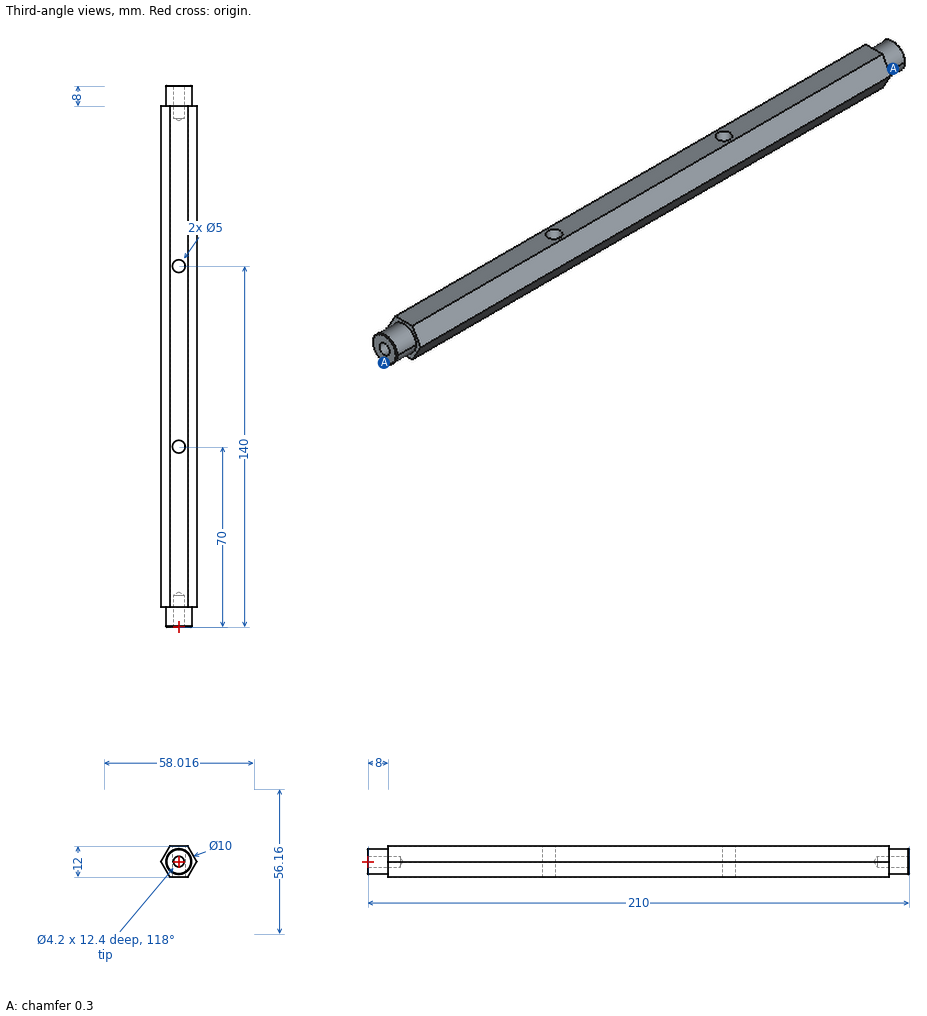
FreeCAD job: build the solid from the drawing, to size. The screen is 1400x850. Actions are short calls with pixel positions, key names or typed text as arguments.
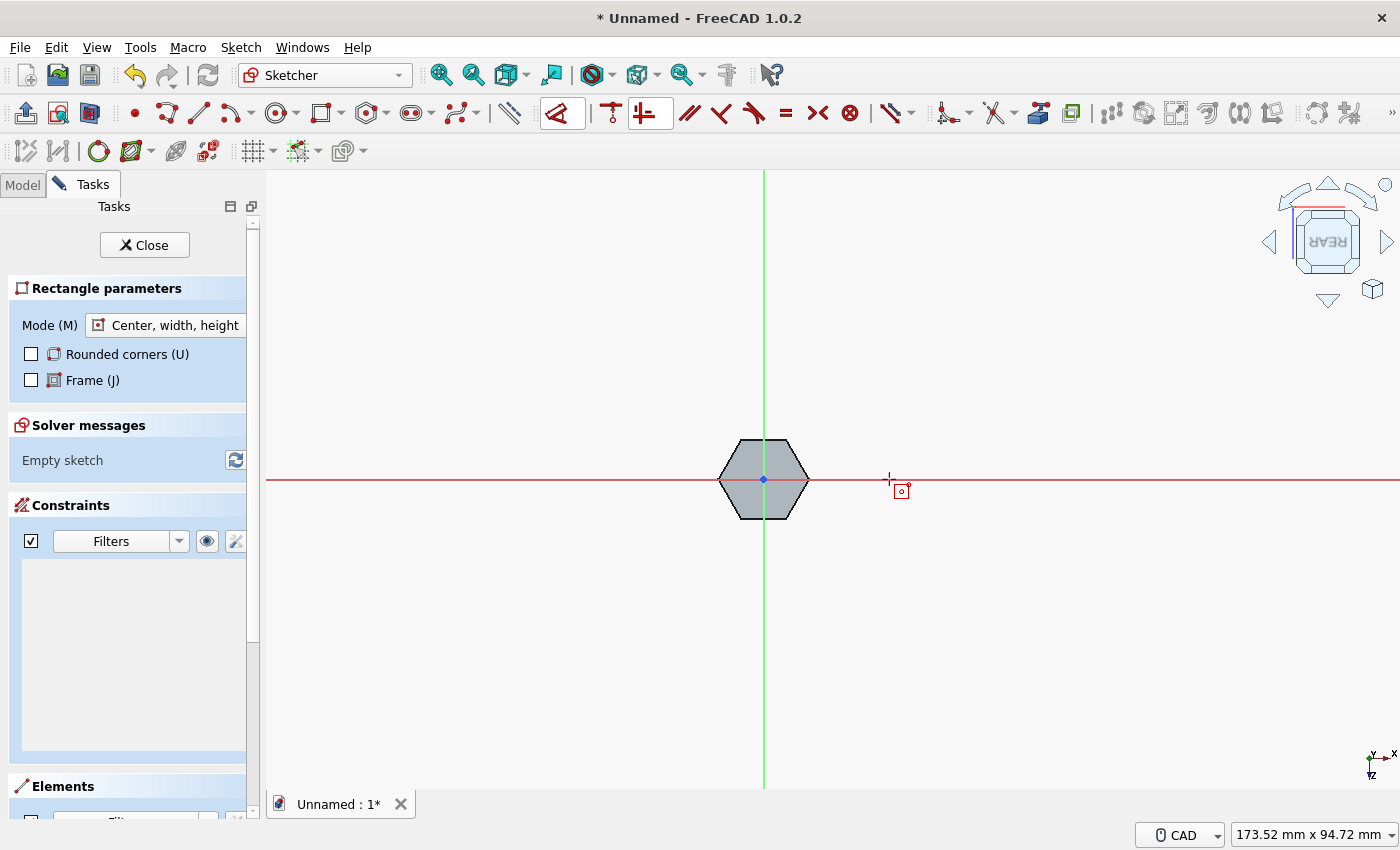
click(764, 479)
click(953, 296)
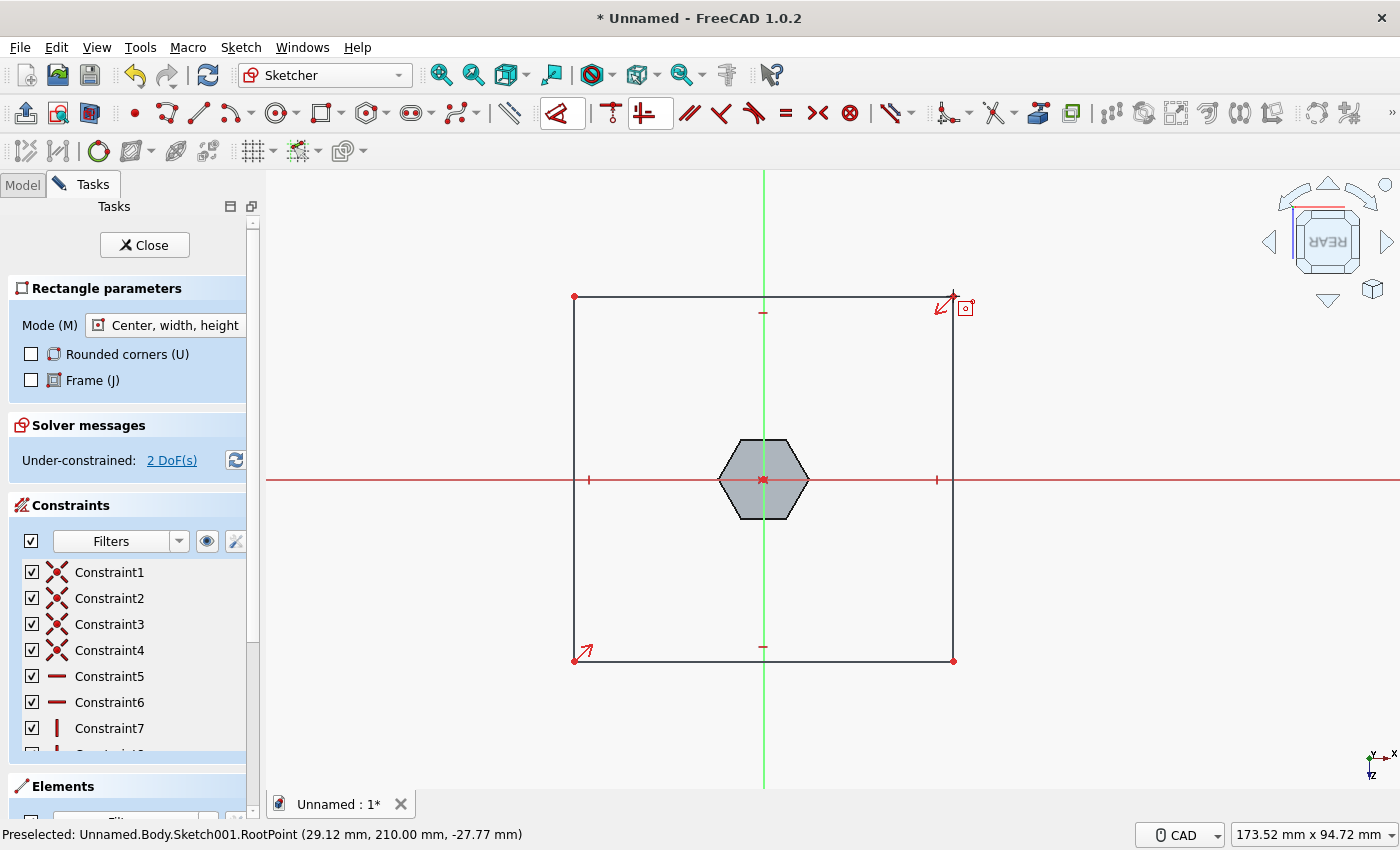
key(g)
key(c)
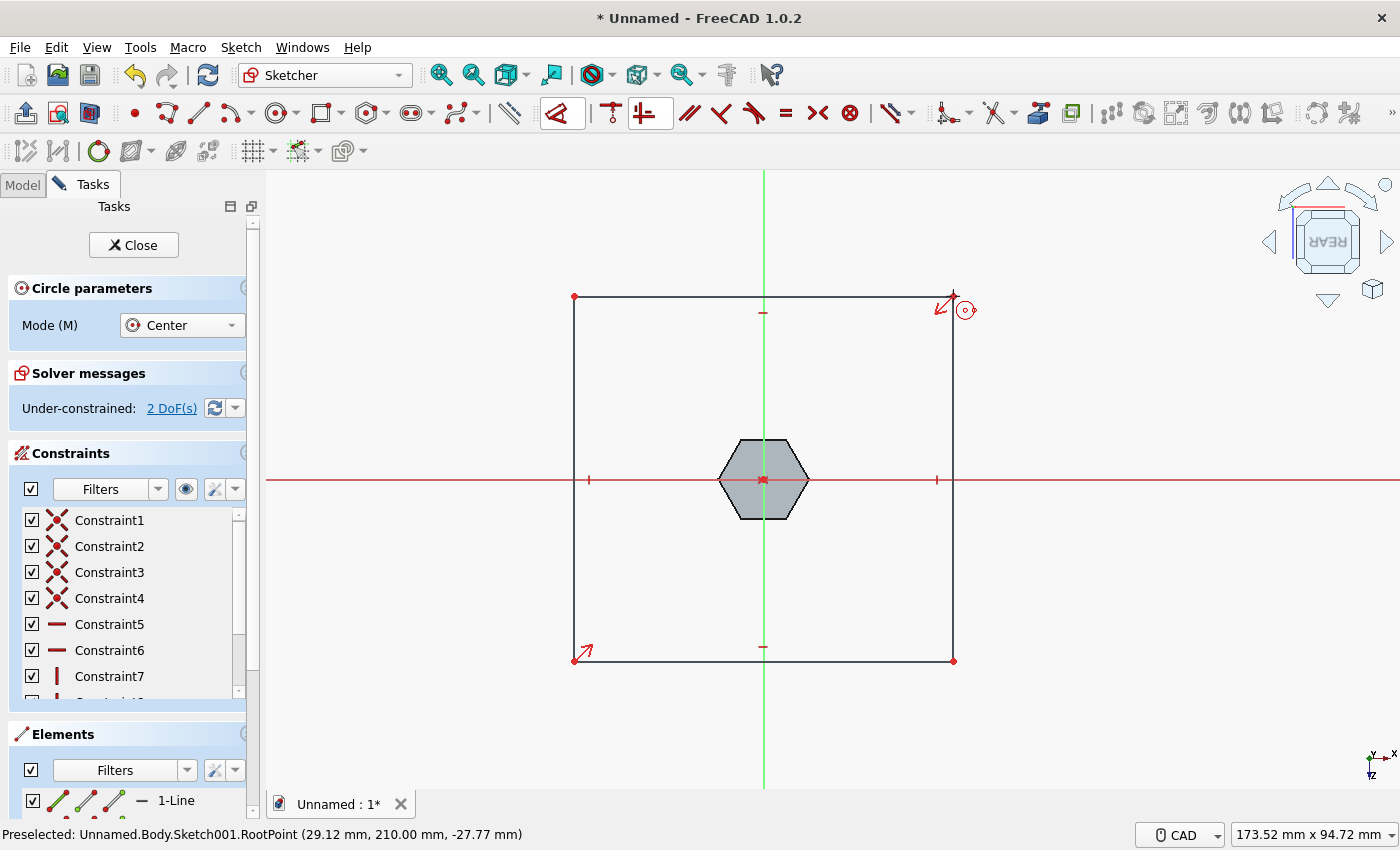
click(764, 479)
click(787, 456)
key(Escape)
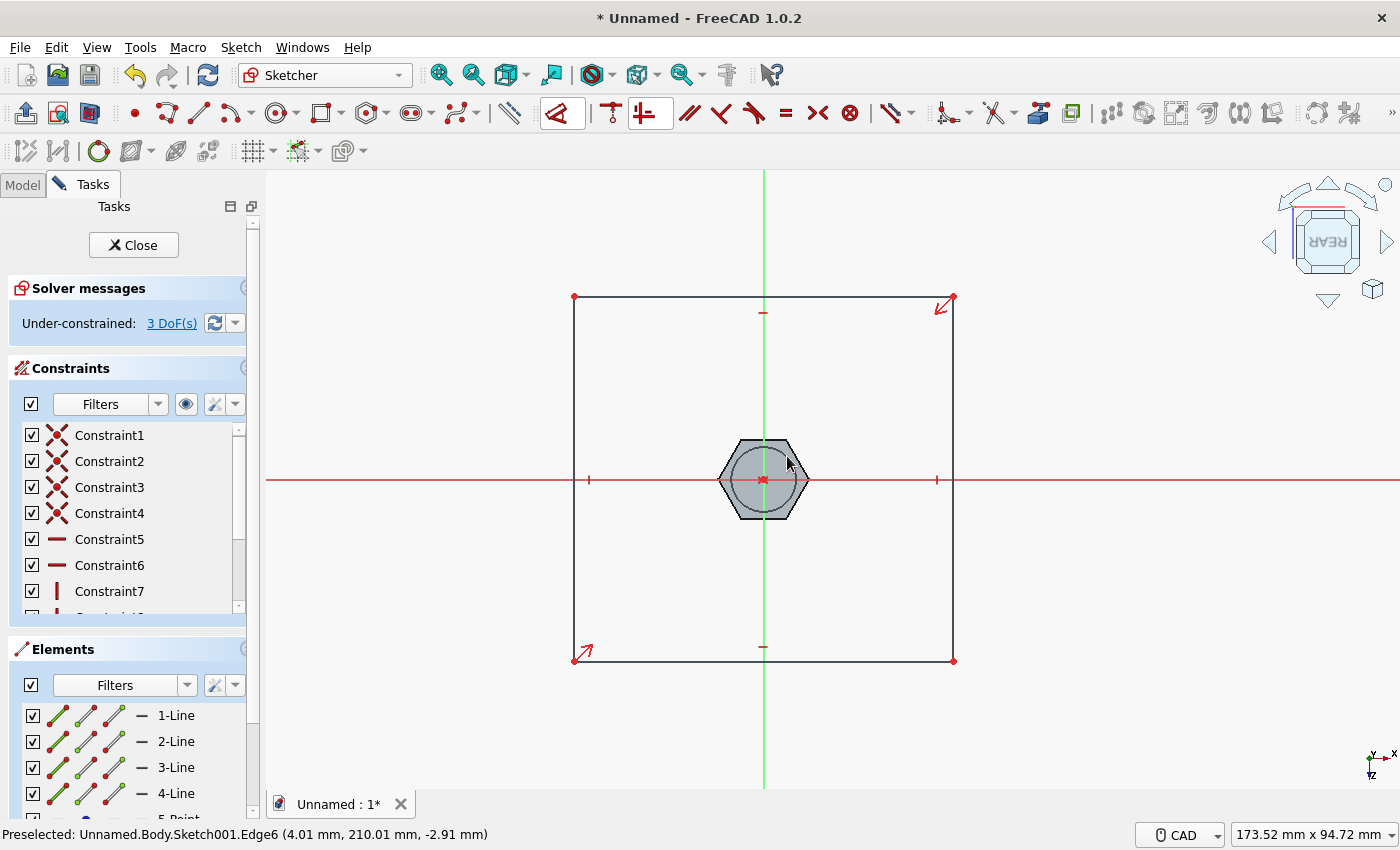
click(787, 457)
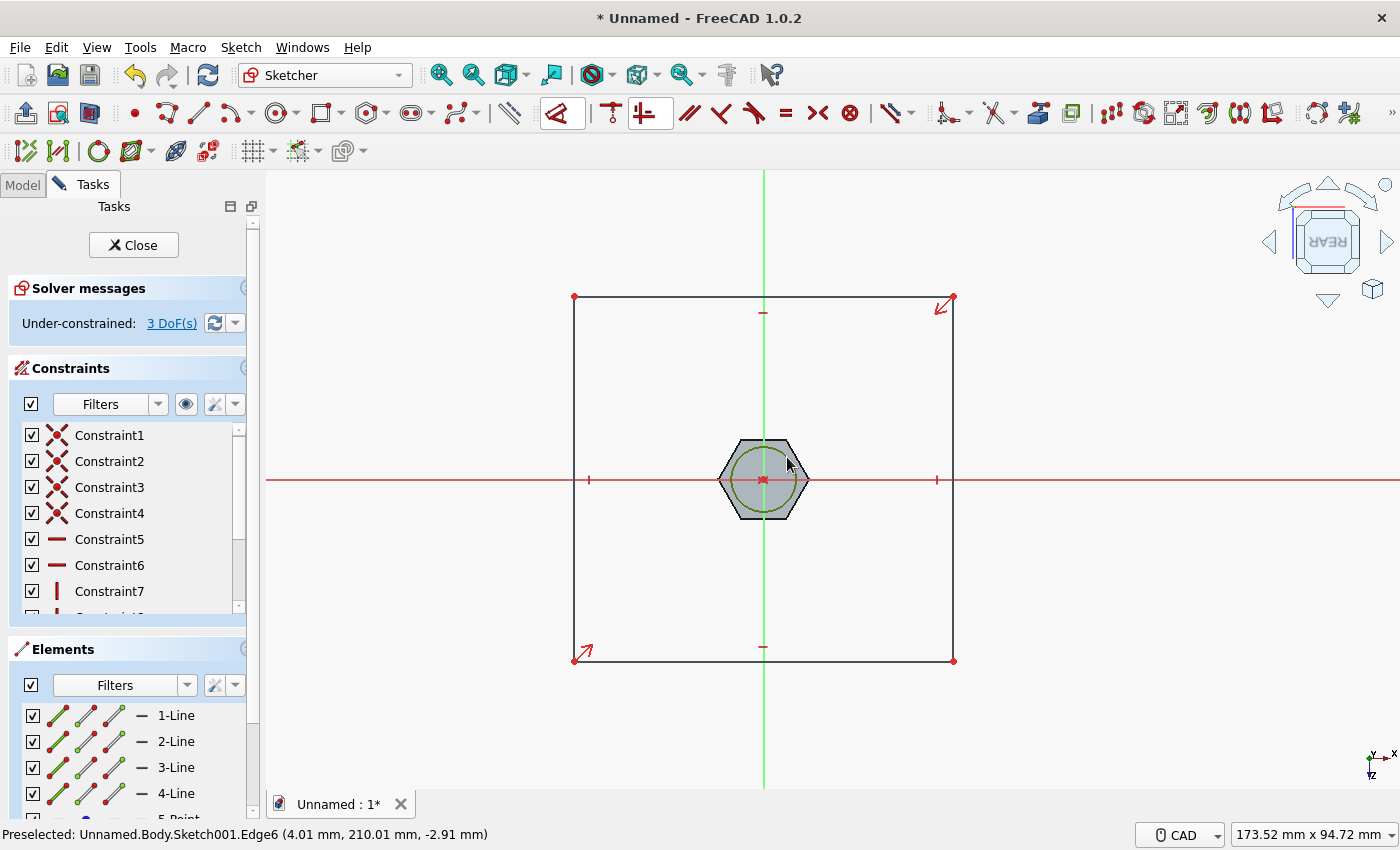
click(580, 114)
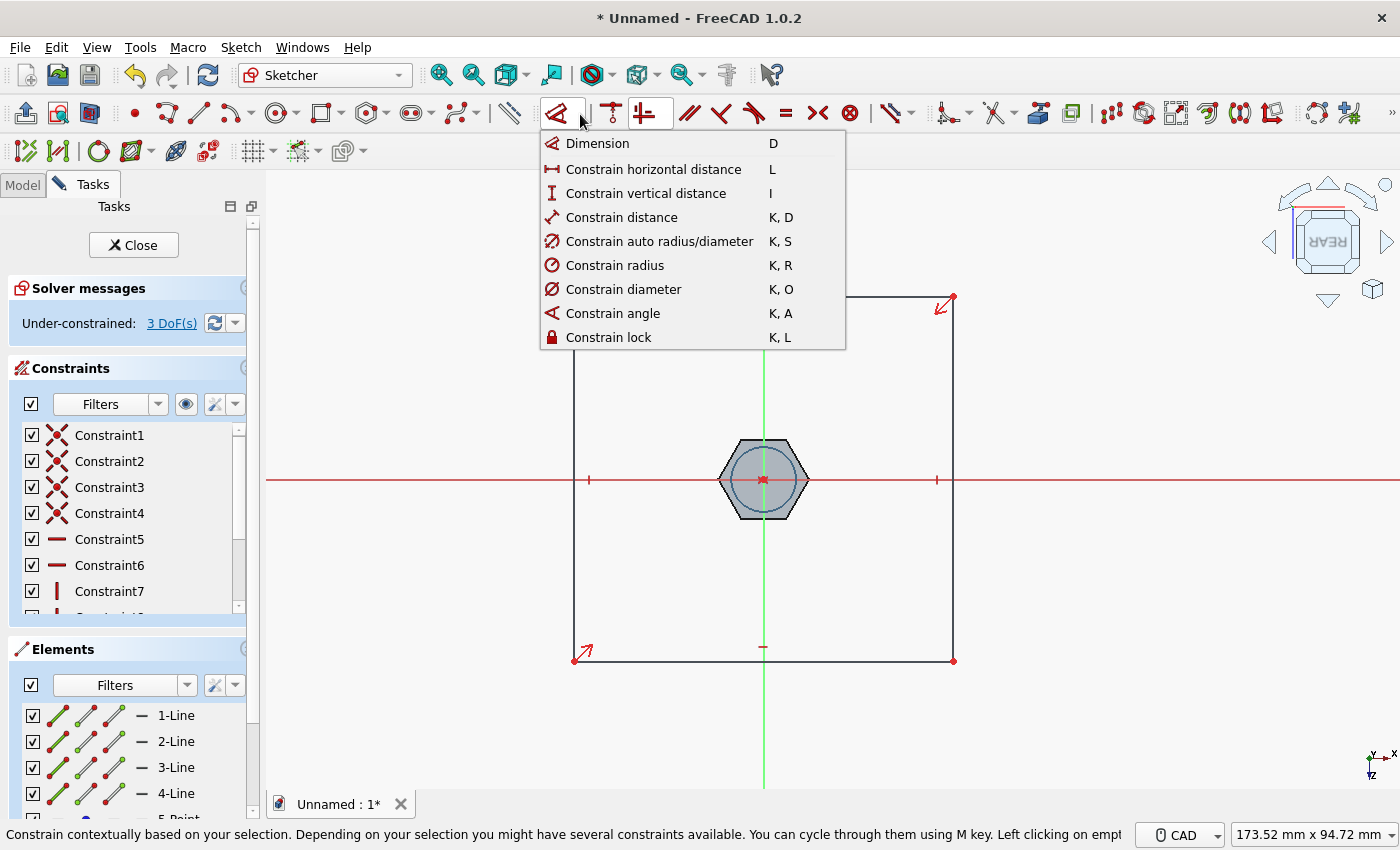
click(693, 289)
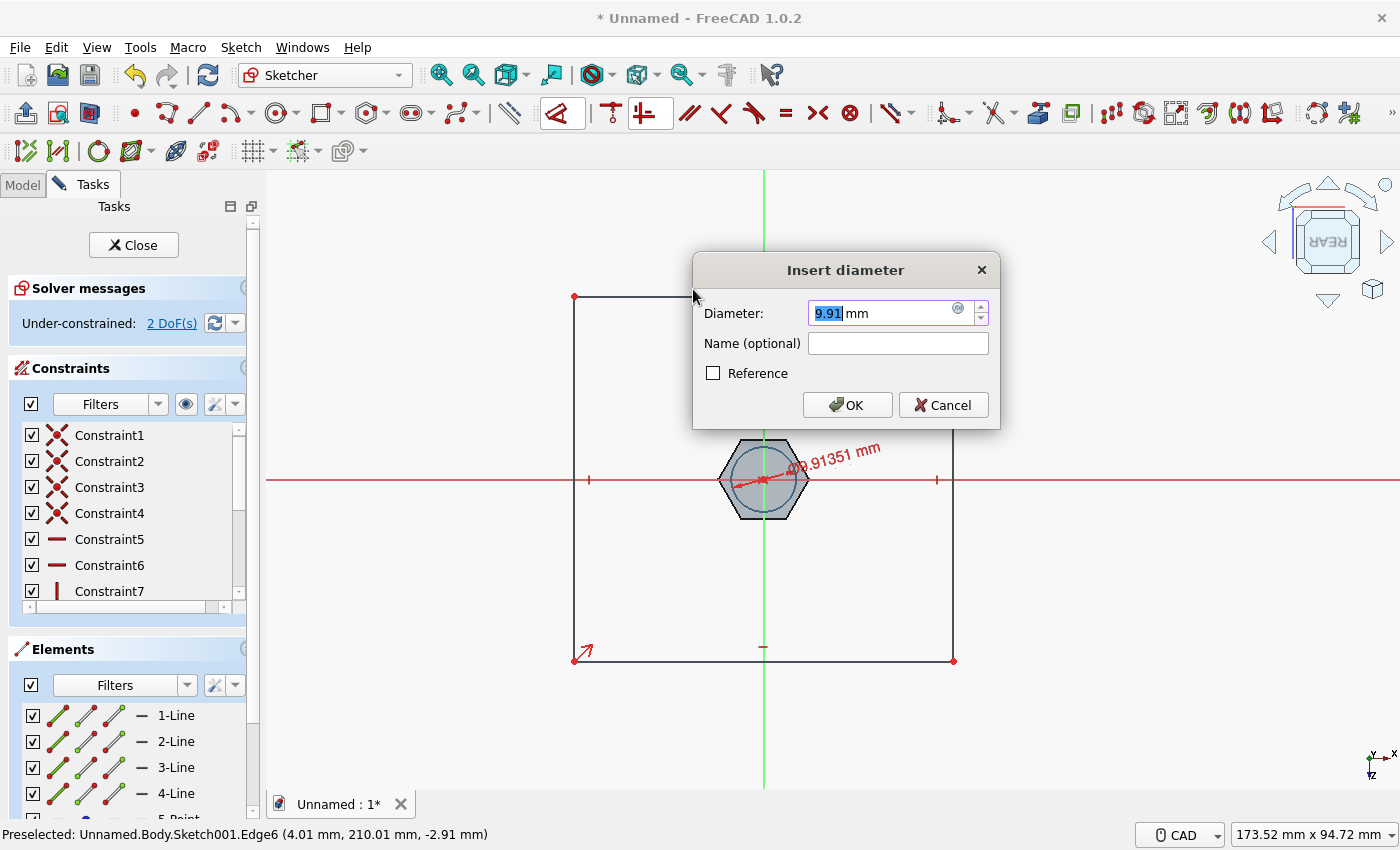
text(10)
key(Return)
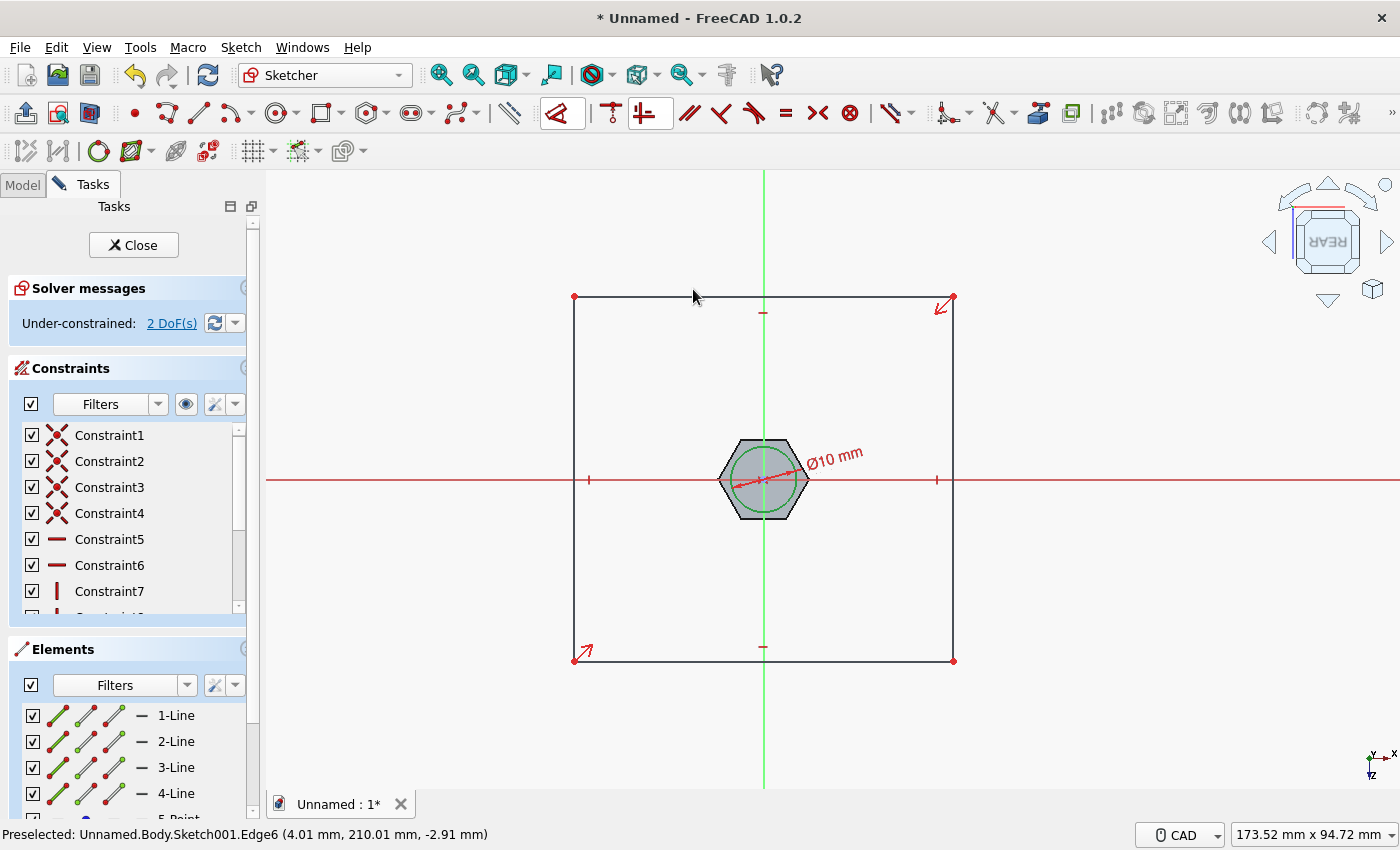
click(953, 552)